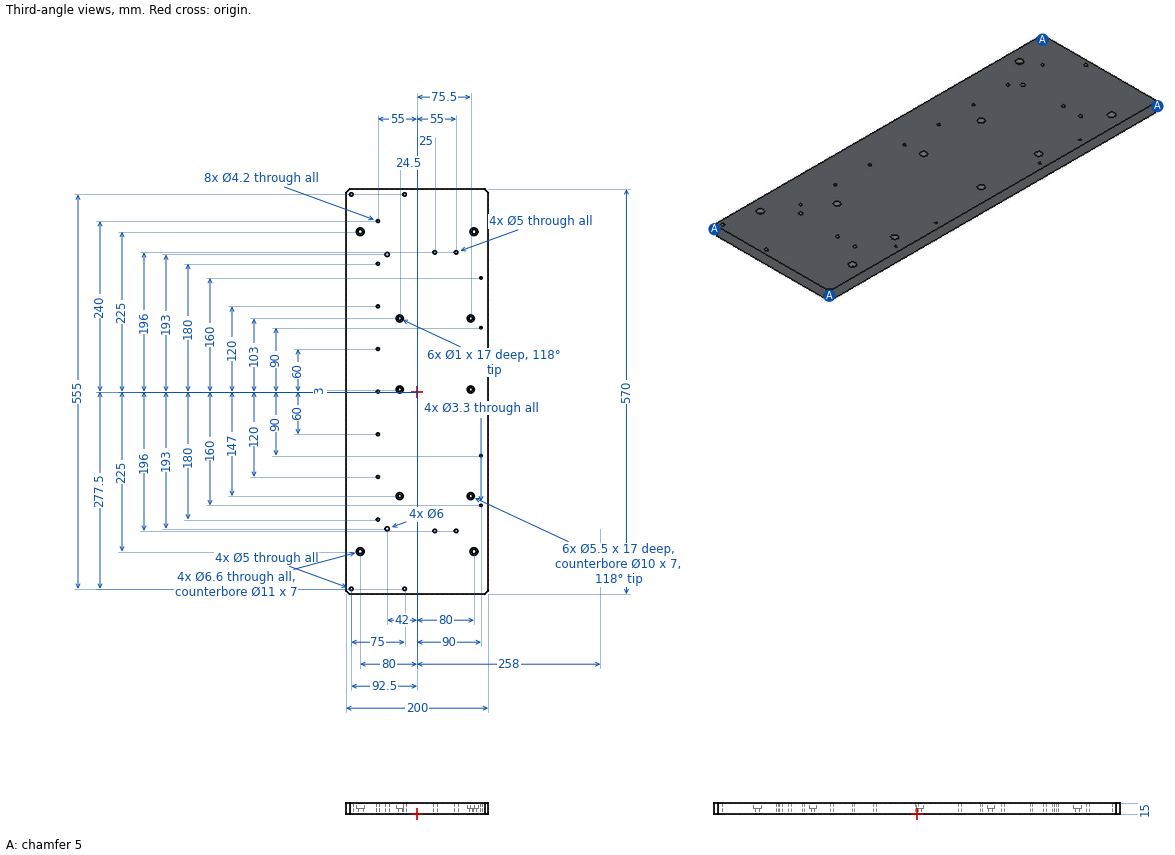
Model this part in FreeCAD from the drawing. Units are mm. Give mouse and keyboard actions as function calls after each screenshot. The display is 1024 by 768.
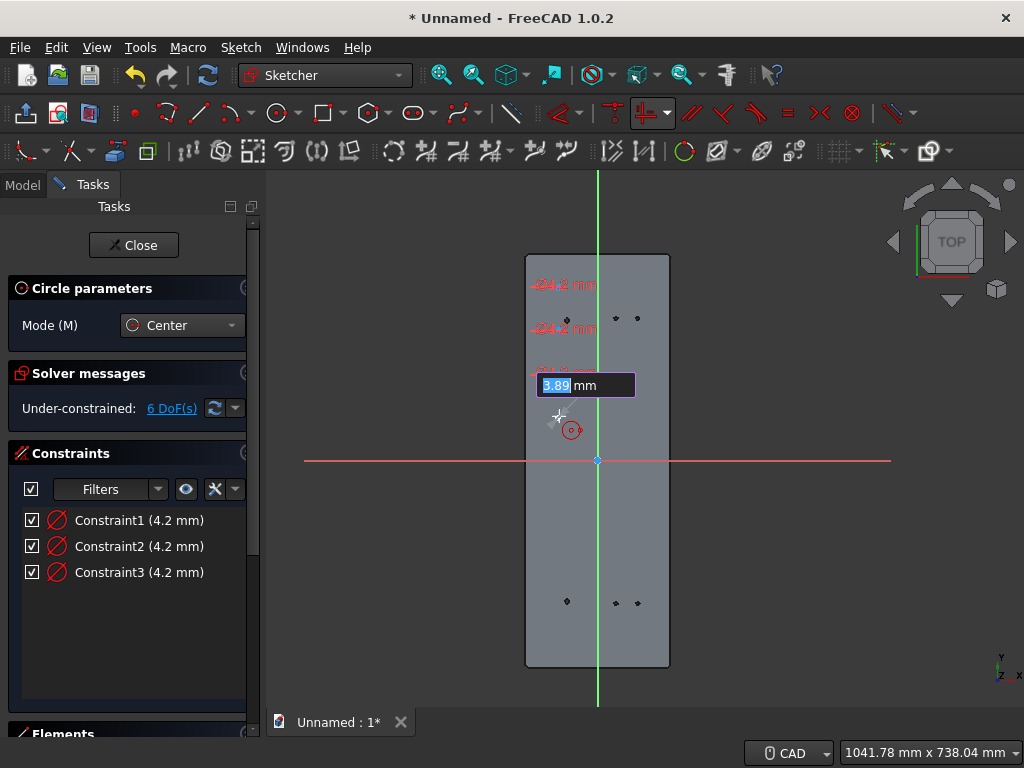
text(4.2)
key(Return)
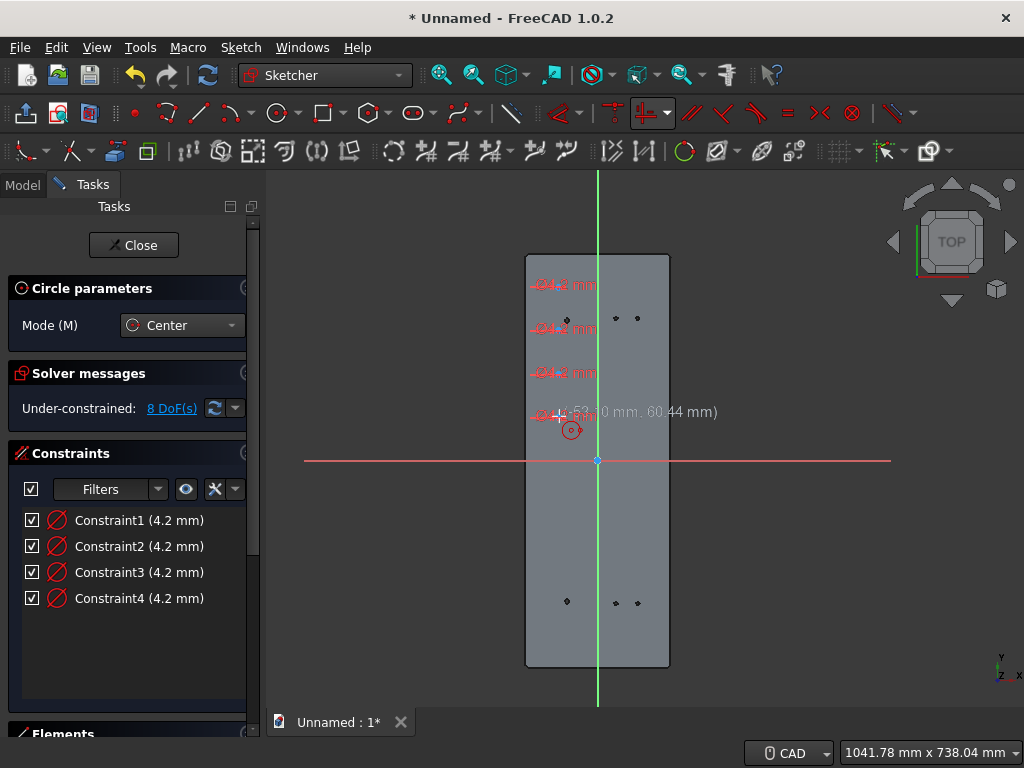
scroll(558, 461, up, 14)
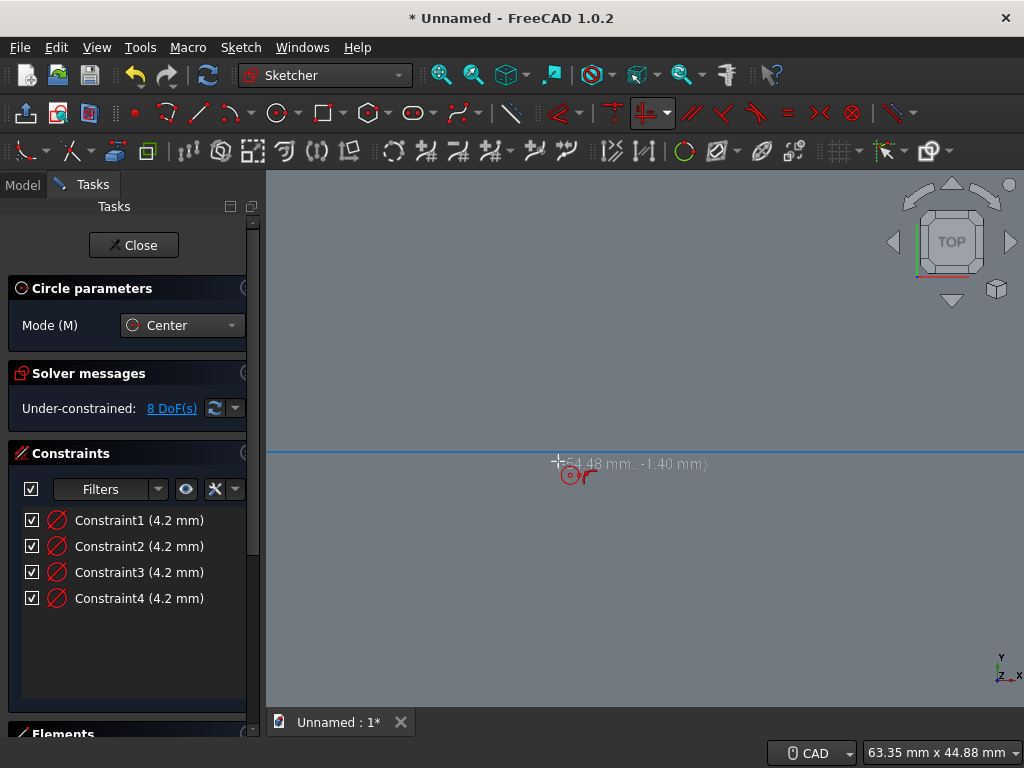
scroll(558, 461, down, 14)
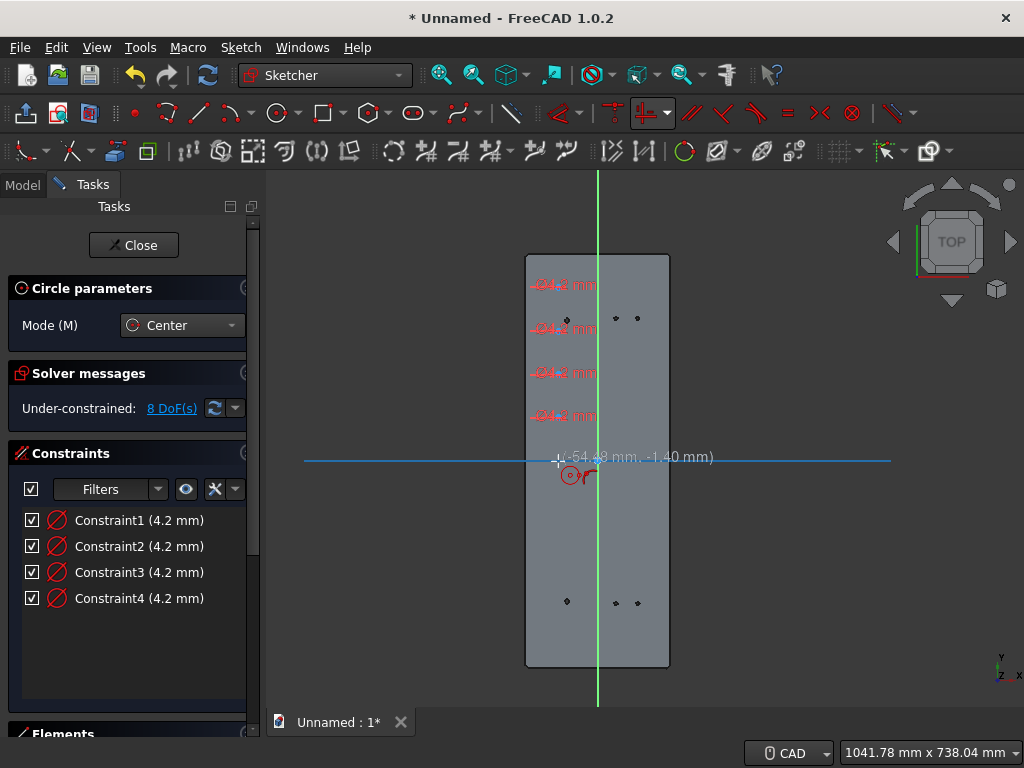
click(558, 461)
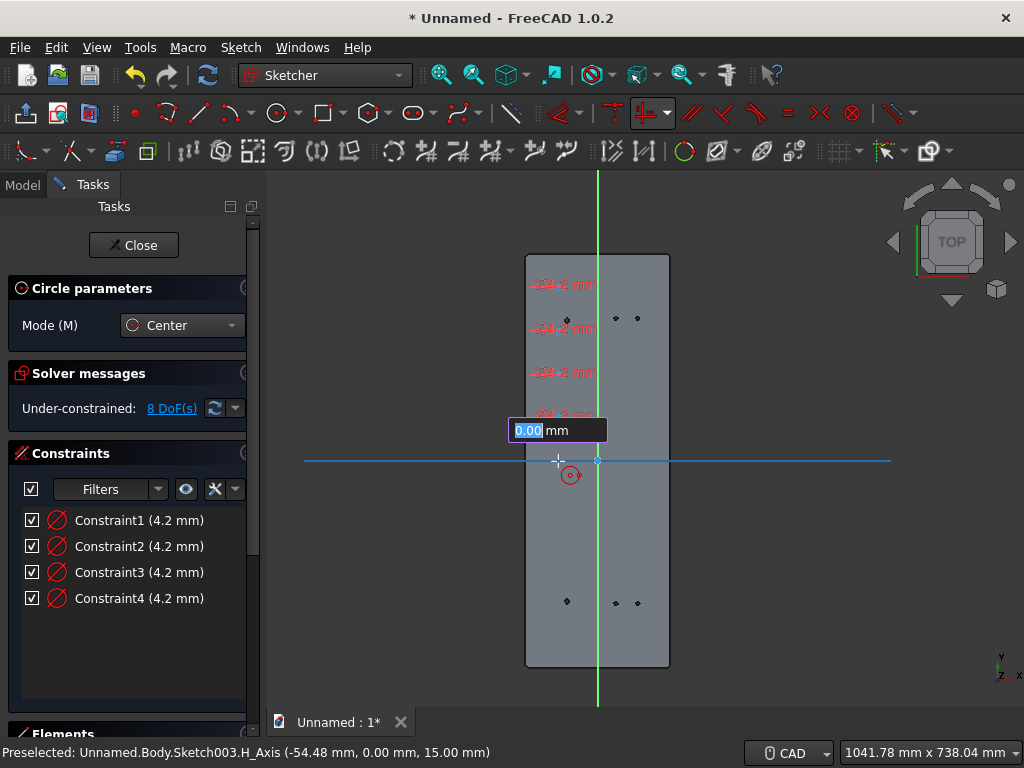
scroll(557, 462, up, 13)
move(554, 461)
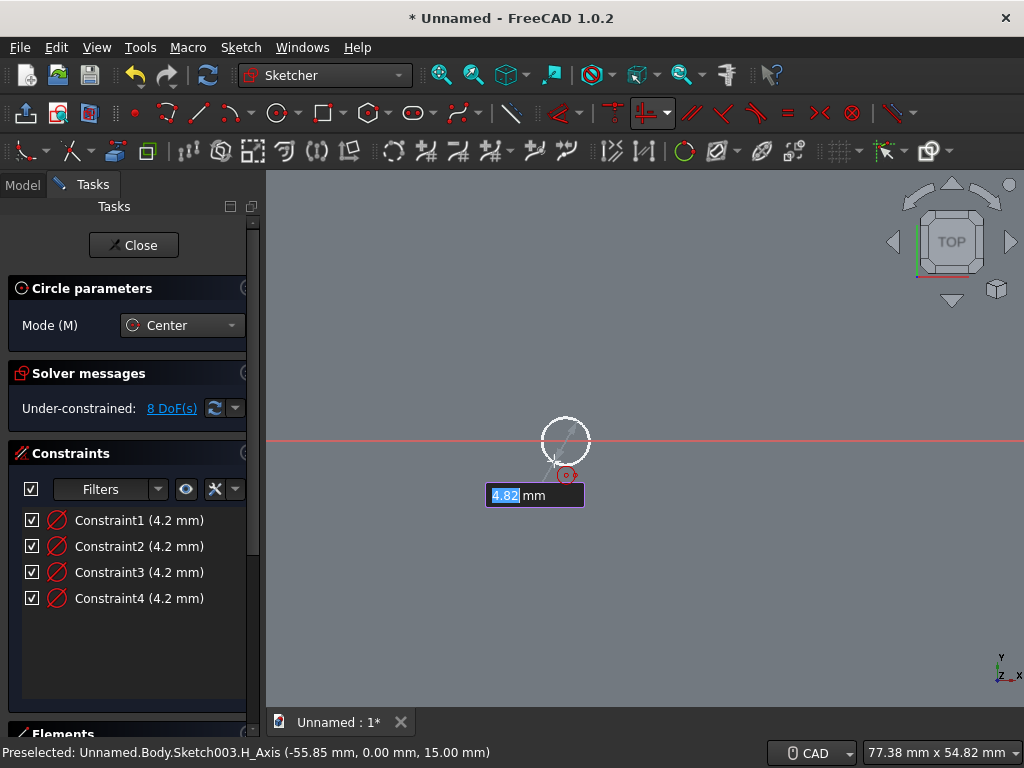
text(4.2)
key(Return)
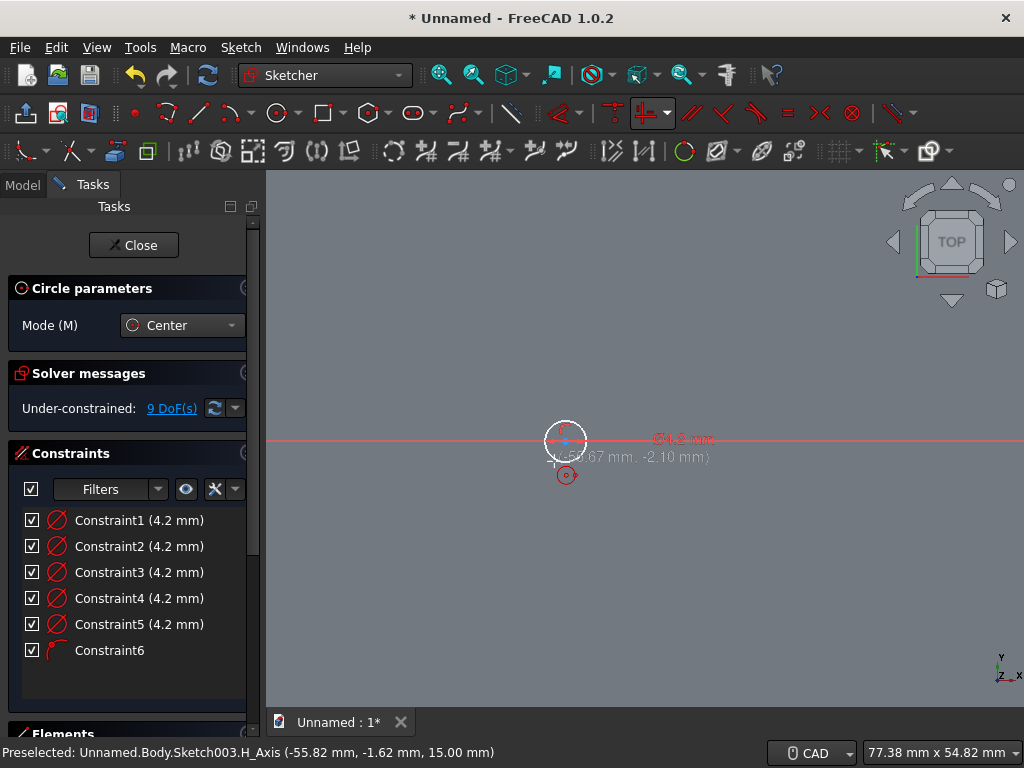
scroll(557, 462, down, 13)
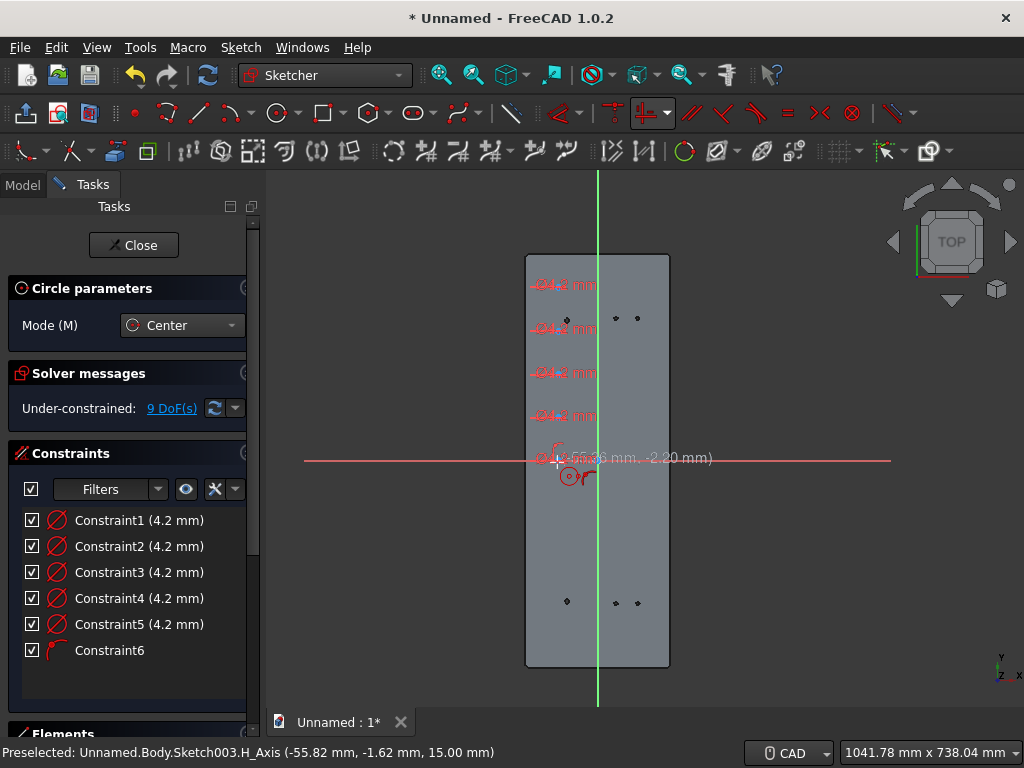
scroll(558, 505, up, 14)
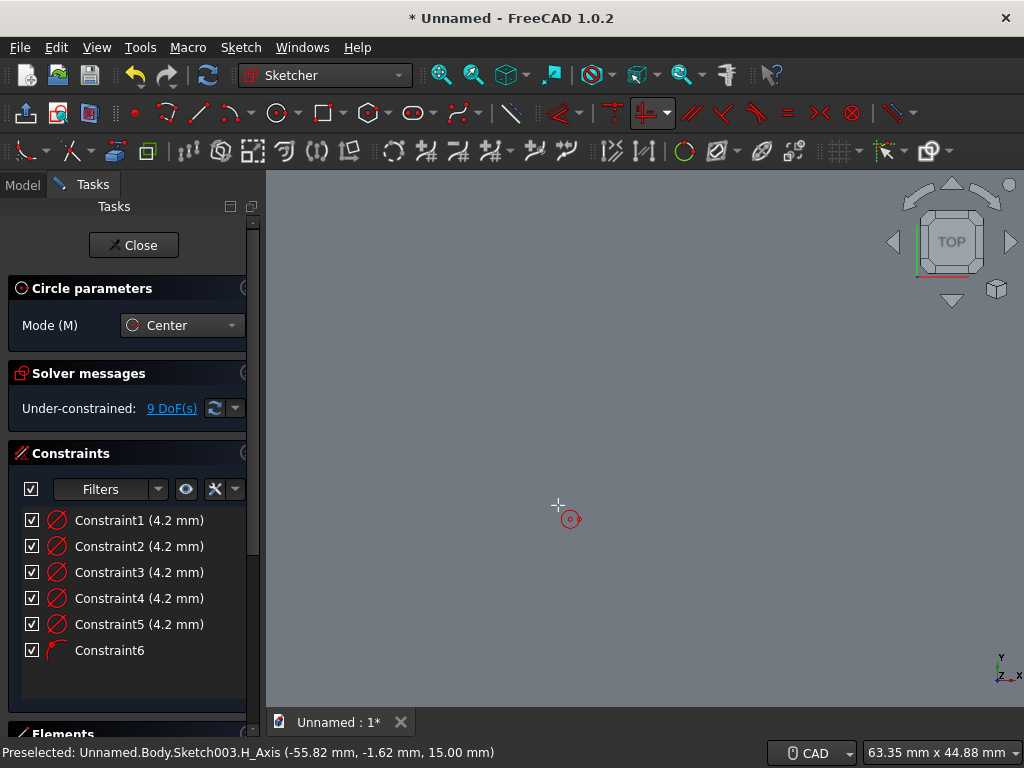
scroll(558, 505, down, 14)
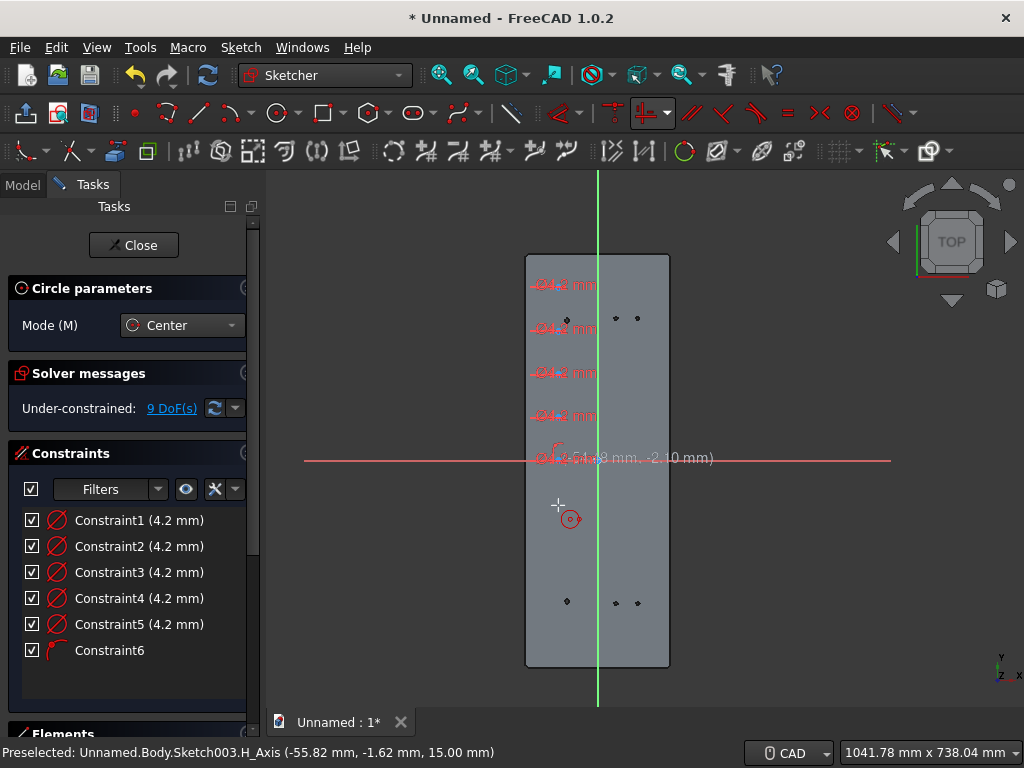
click(558, 505)
move(559, 504)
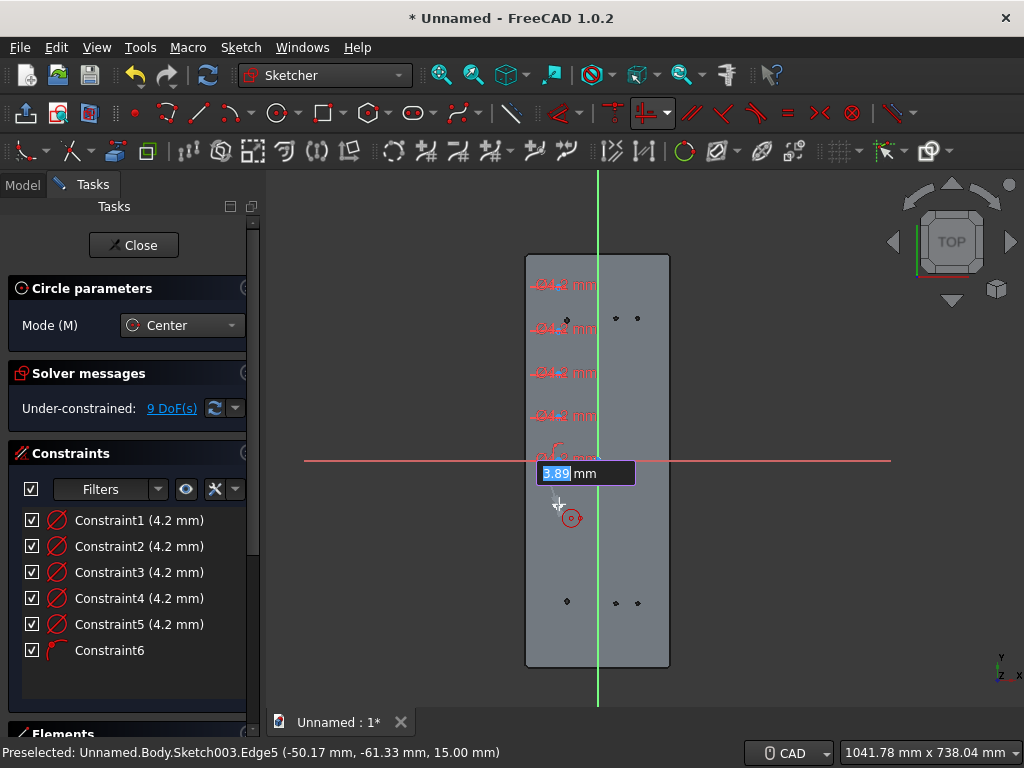
text(4.2)
key(Return)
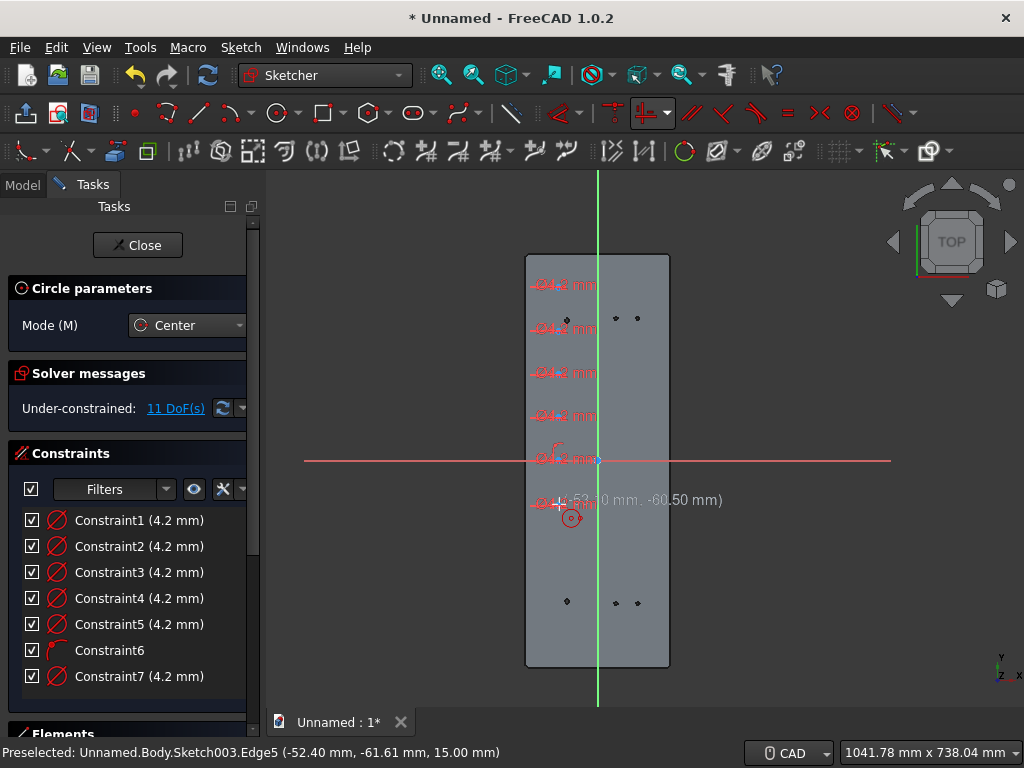
scroll(558, 548, up, 14)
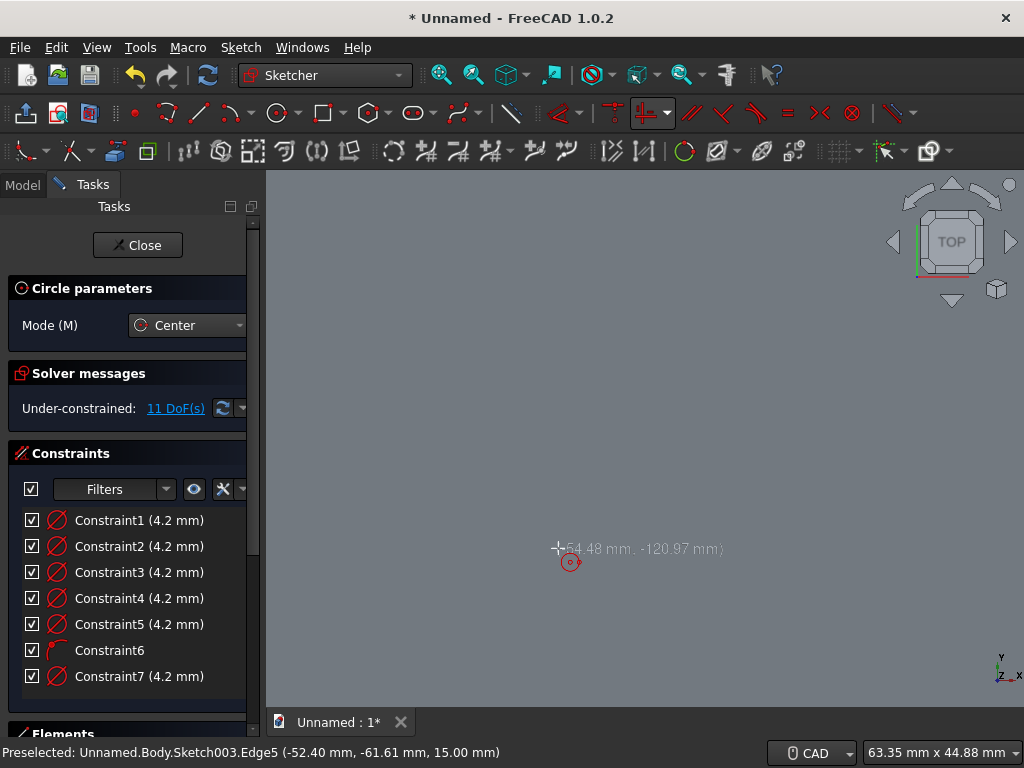
scroll(558, 548, down, 14)